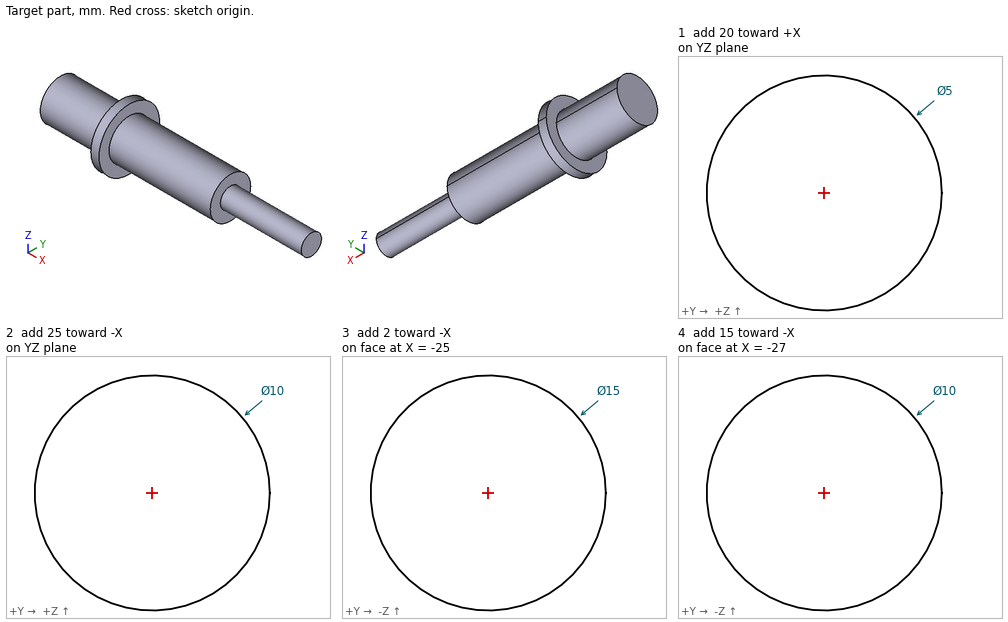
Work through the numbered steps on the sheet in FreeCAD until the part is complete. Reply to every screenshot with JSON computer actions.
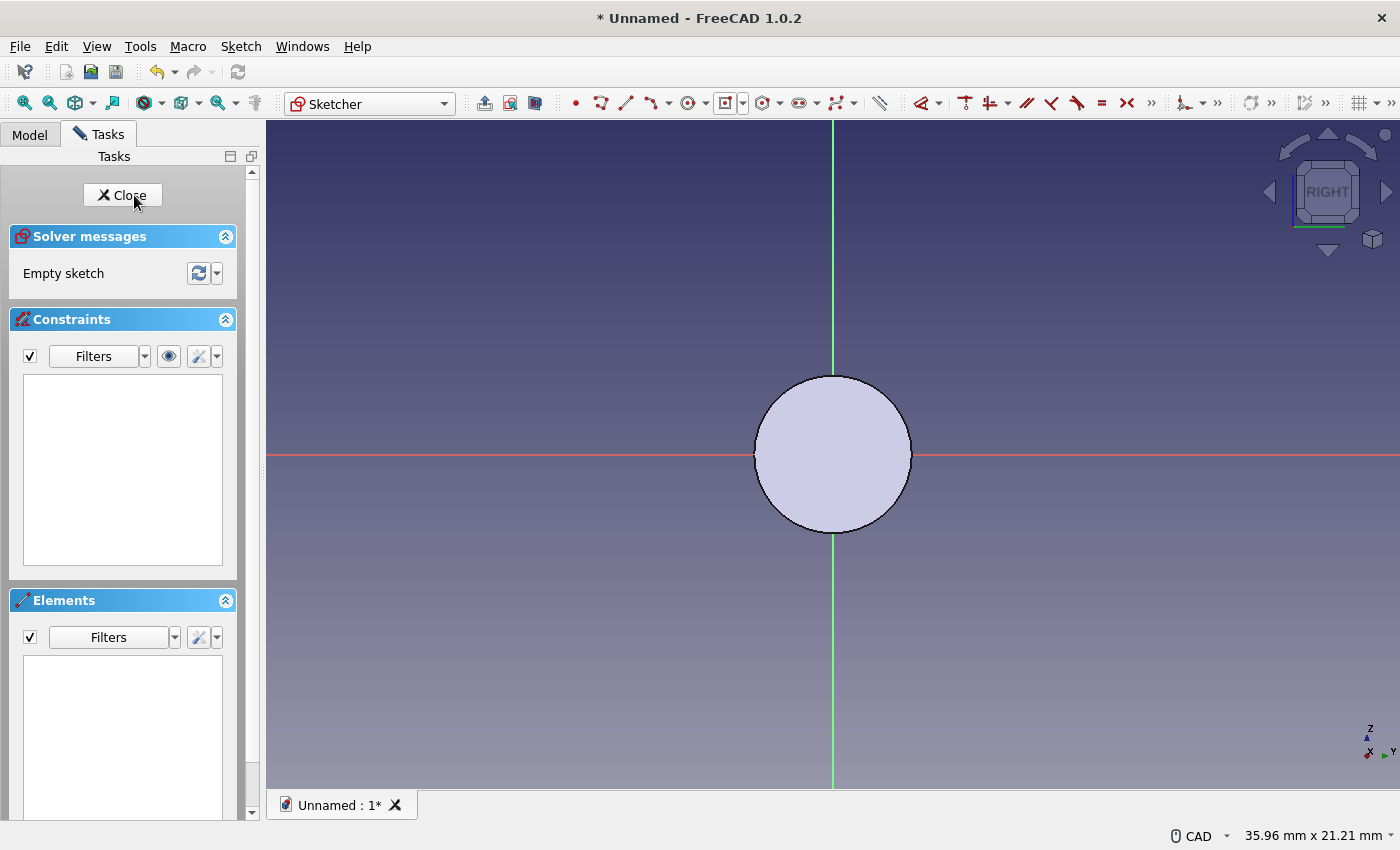
{"action": "key", "text": "q s"}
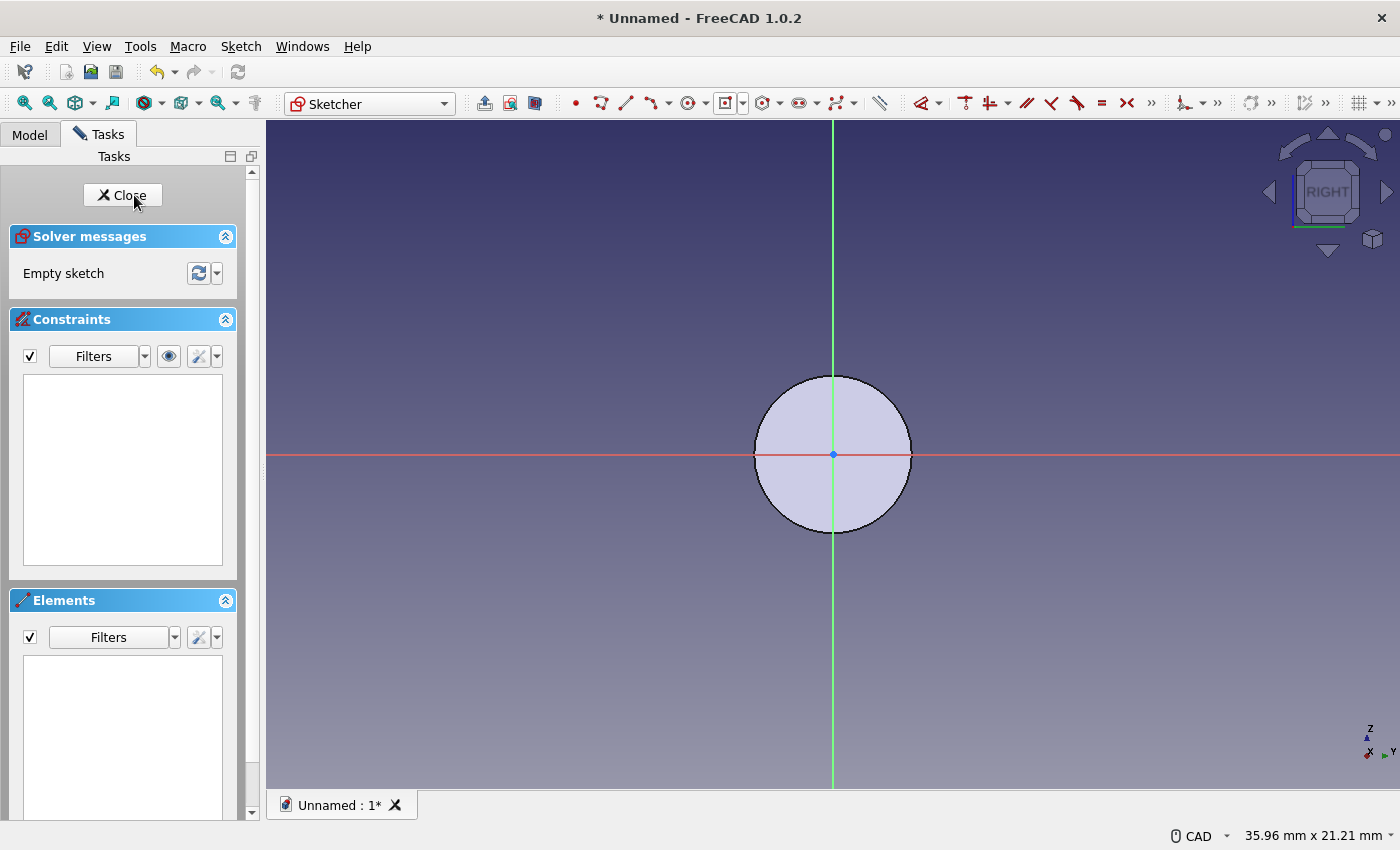
{"action": "scroll", "coordinate": [972, 455], "scroll_direction": "up", "scroll_amount": 2}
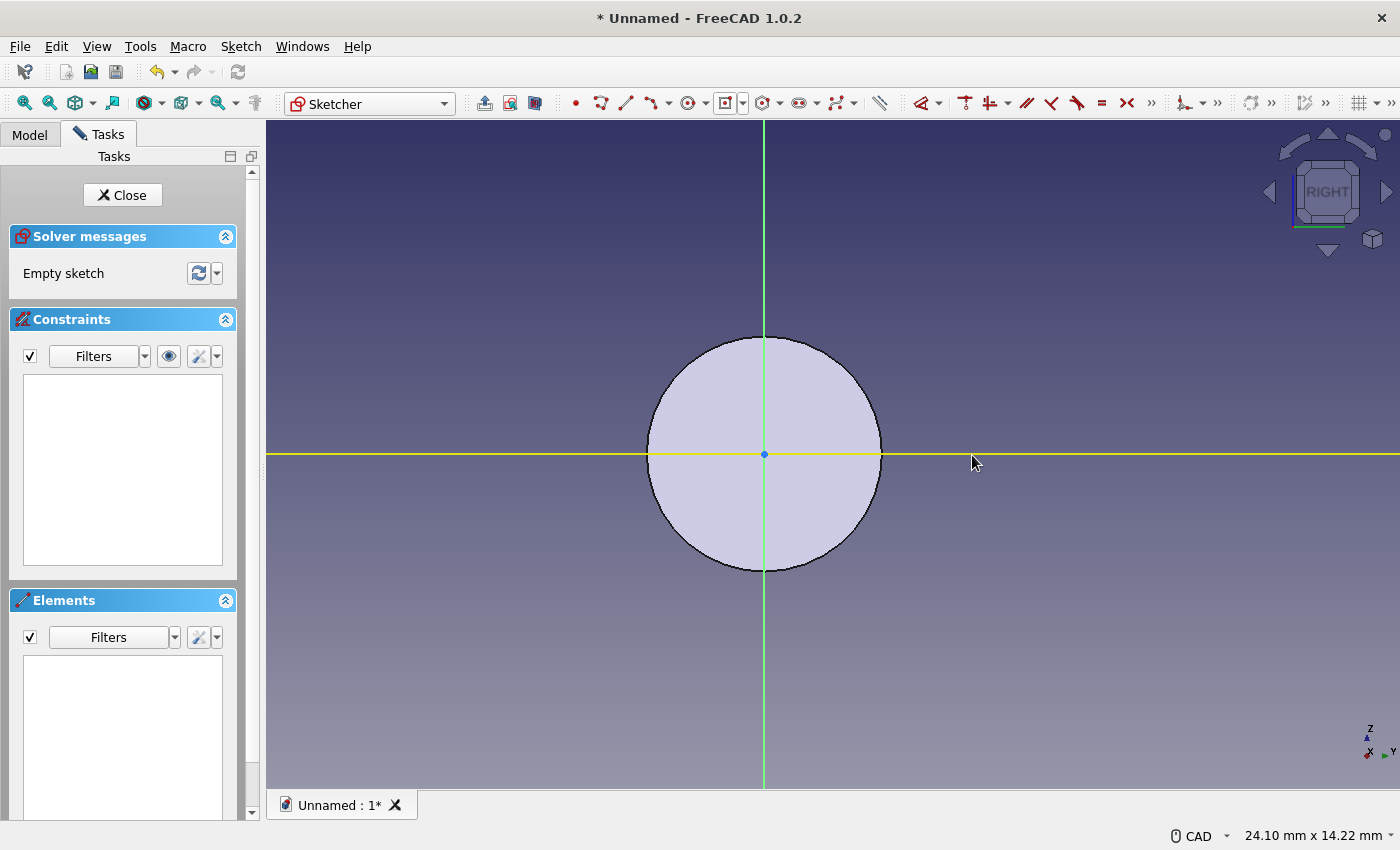
{"action": "left_click", "coordinate": [688, 104]}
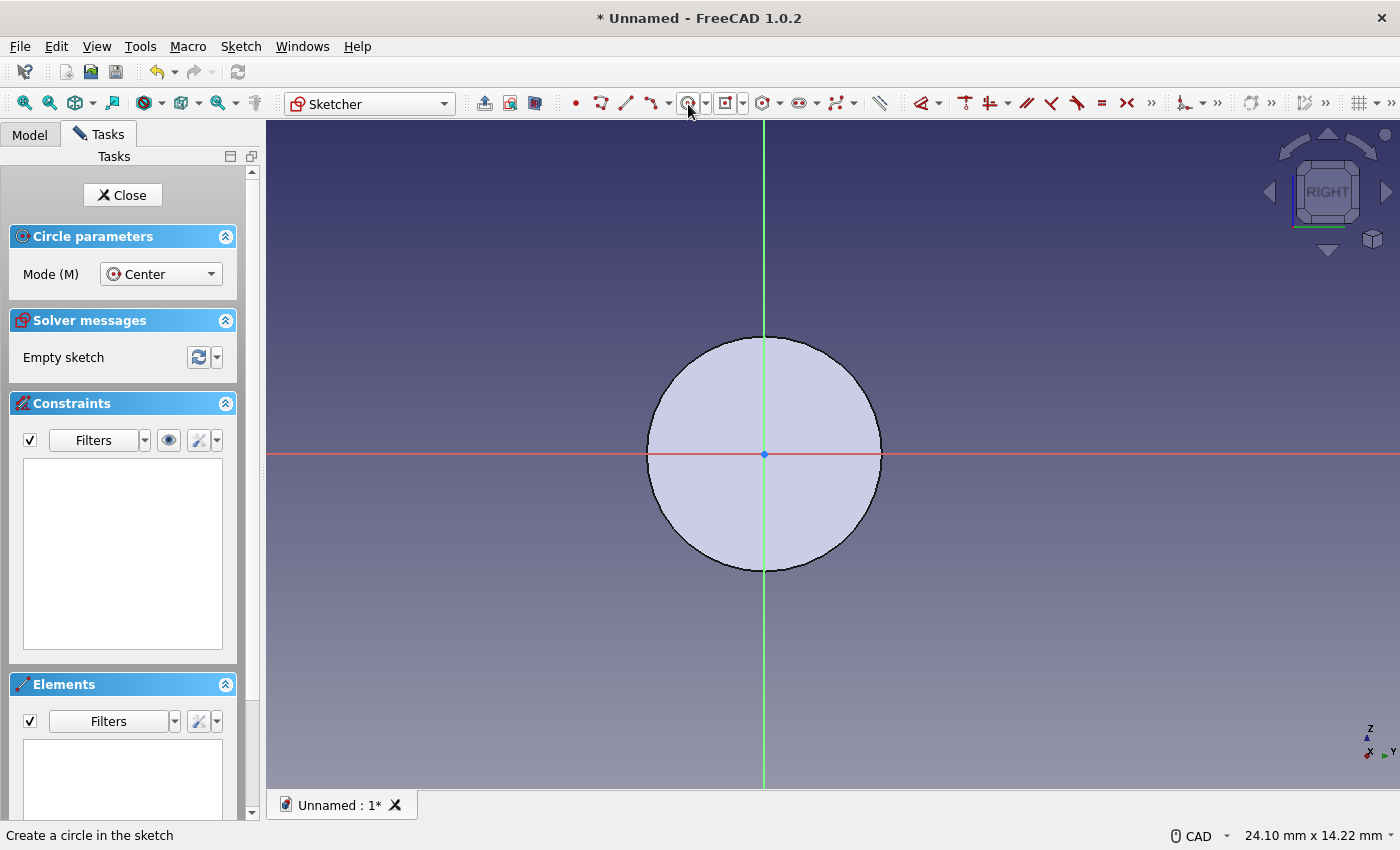
{"action": "left_click", "coordinate": [764, 454]}
{"action": "left_click", "coordinate": [931, 288]}
{"action": "key", "text": "Escape"}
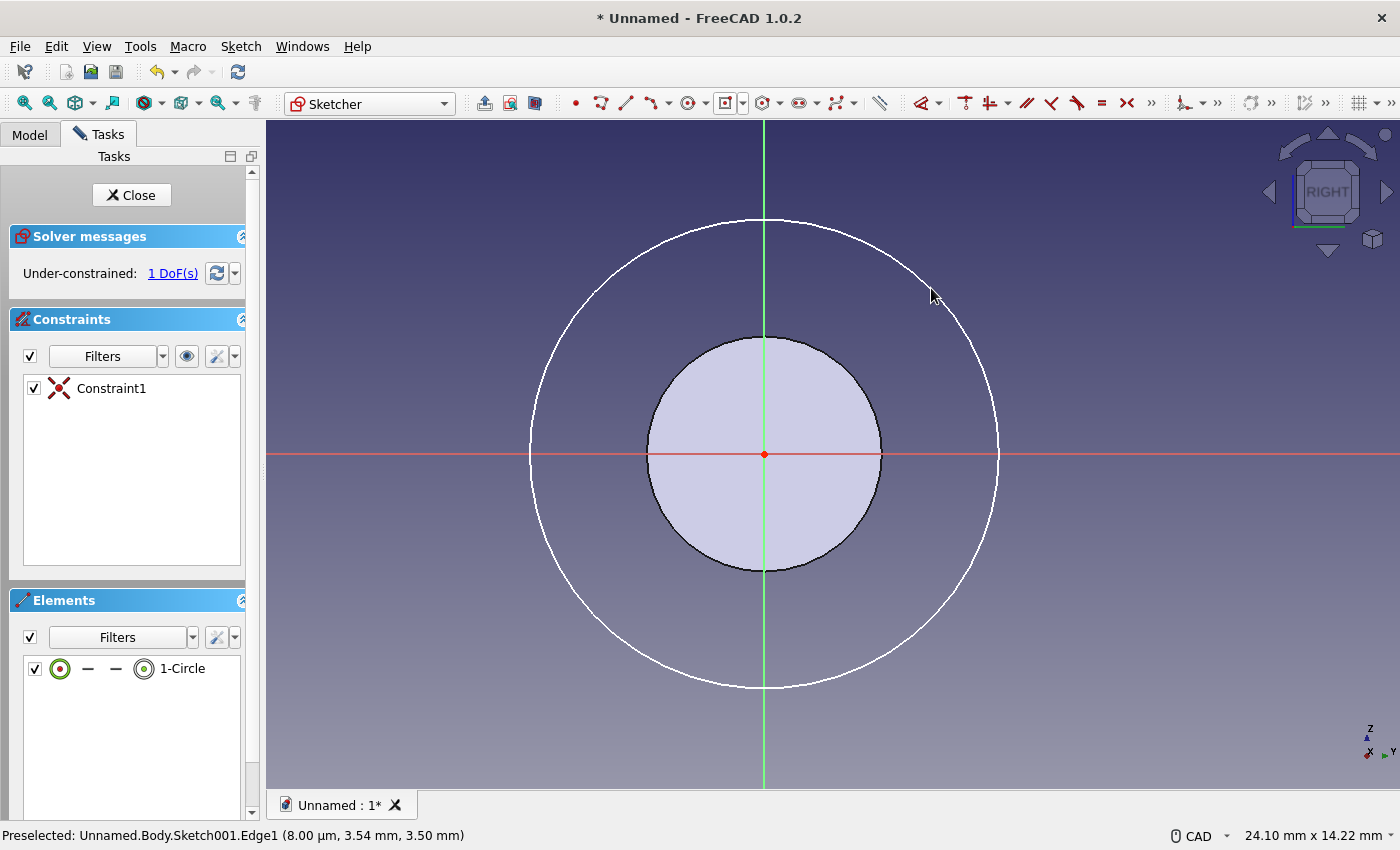
{"action": "key", "text": "d"}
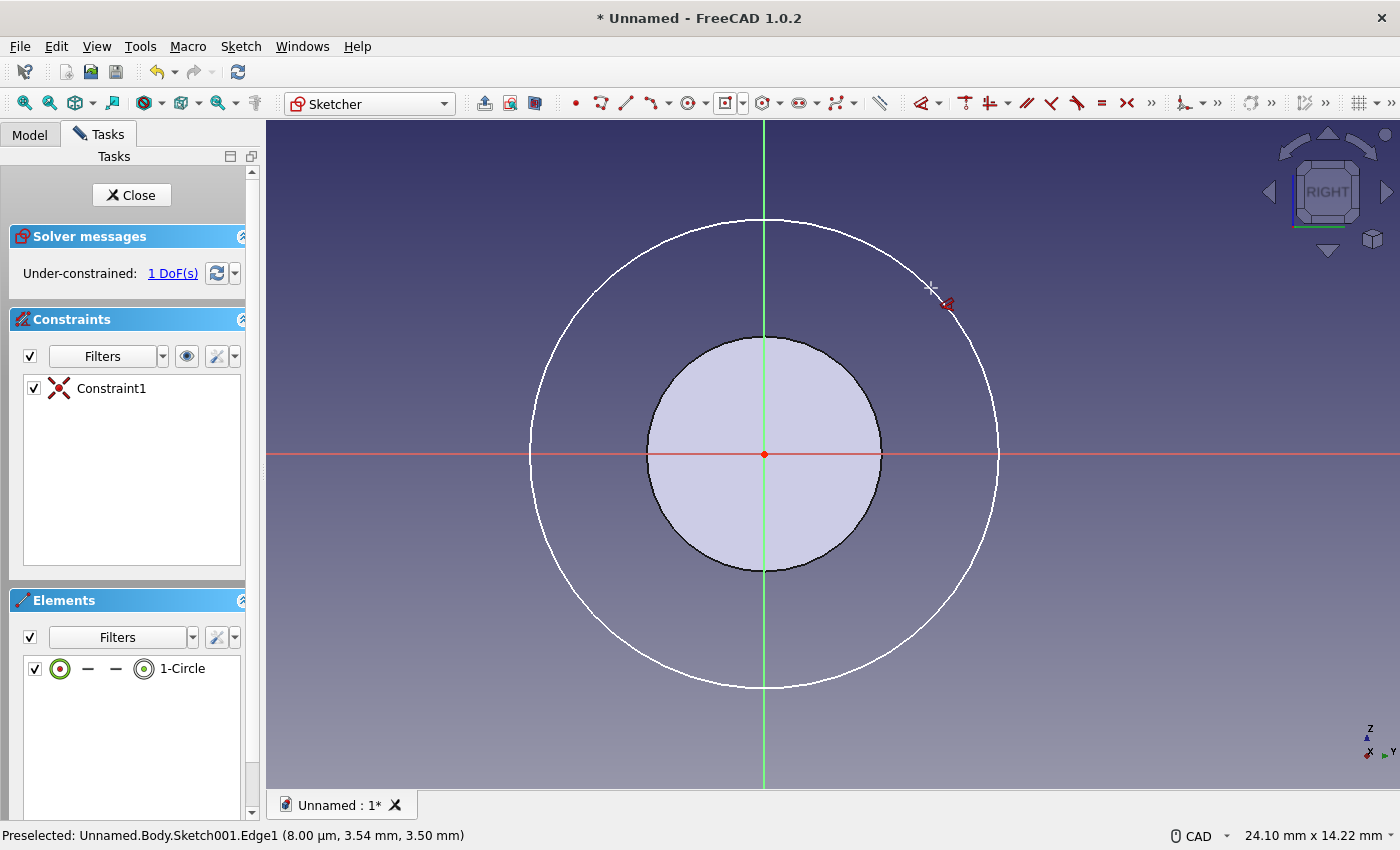
{"action": "left_click", "coordinate": [930, 288]}
{"action": "left_click", "coordinate": [953, 265]}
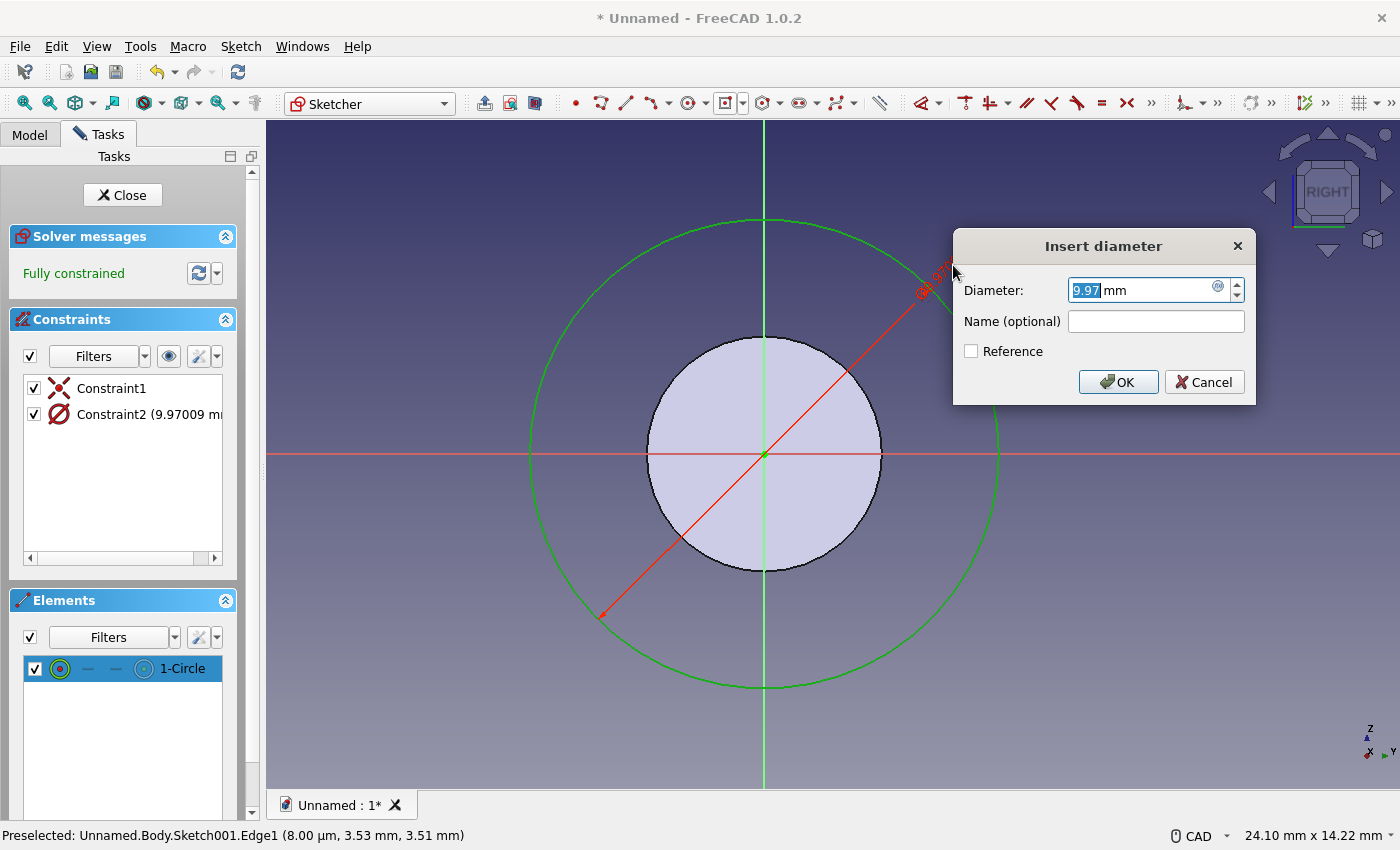
{"action": "type", "text": "10"}
{"action": "key", "text": "Return"}
{"action": "key", "text": "Escape"}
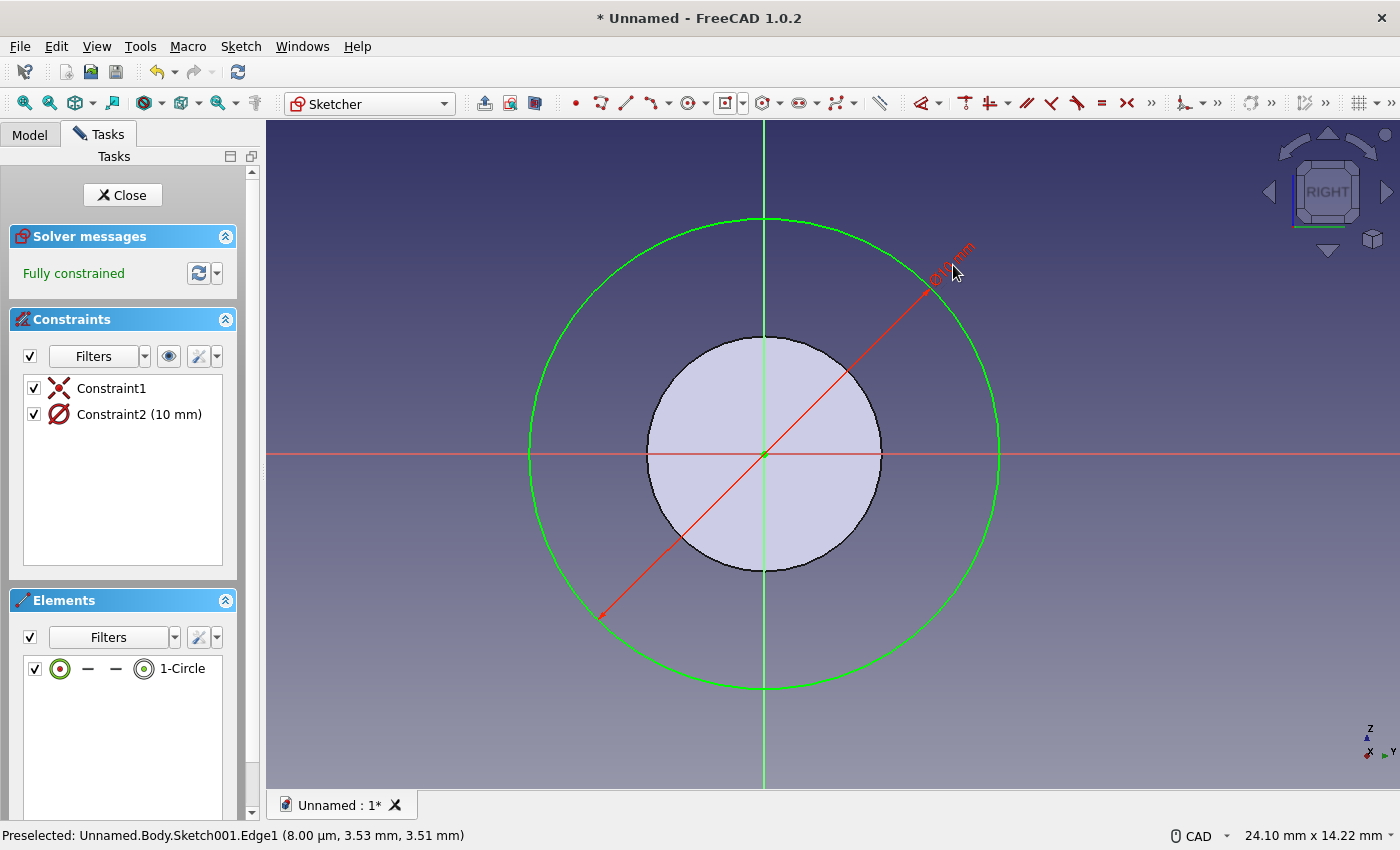
{"action": "left_click", "coordinate": [123, 195]}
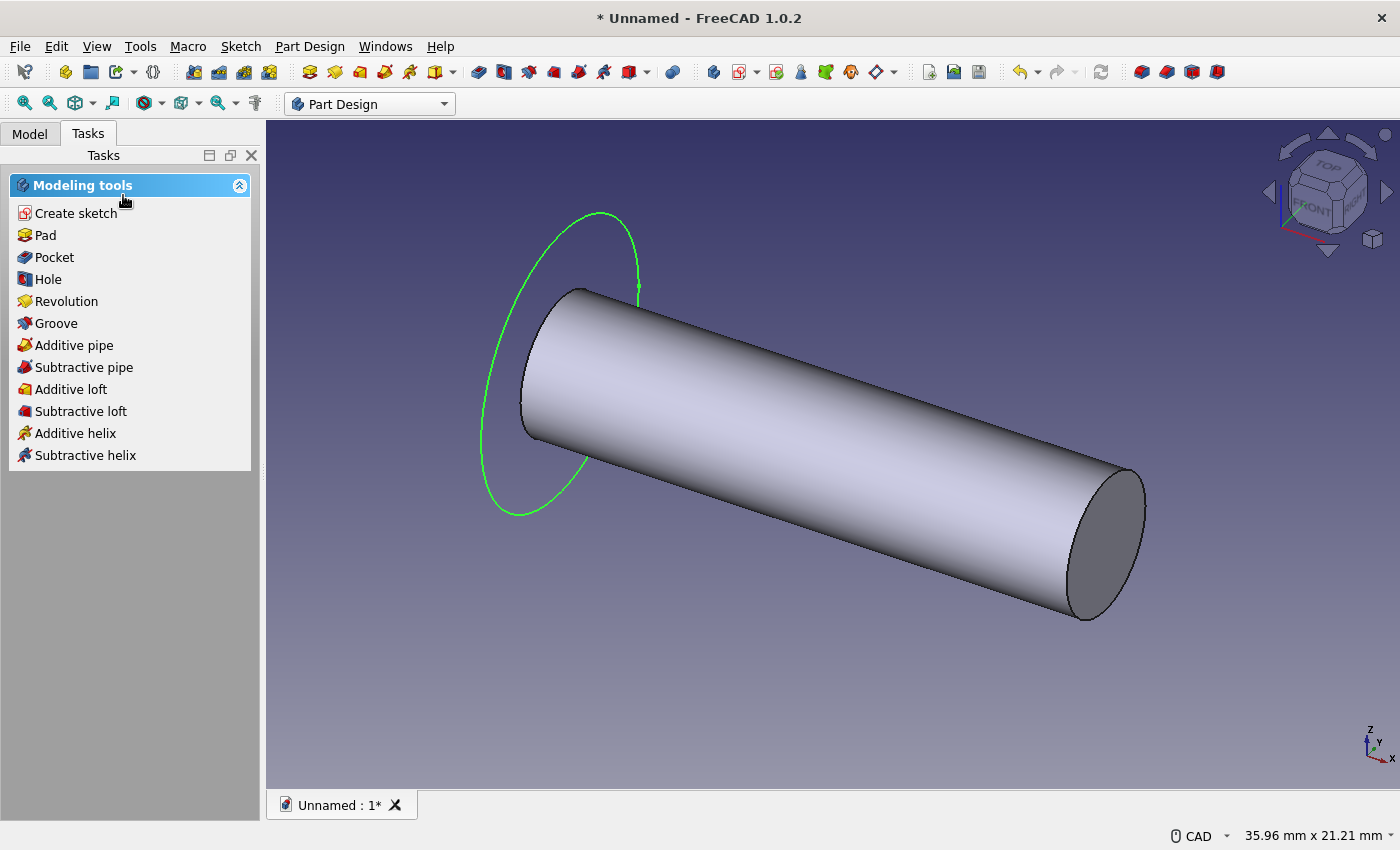
{"action": "left_click", "coordinate": [310, 72]}